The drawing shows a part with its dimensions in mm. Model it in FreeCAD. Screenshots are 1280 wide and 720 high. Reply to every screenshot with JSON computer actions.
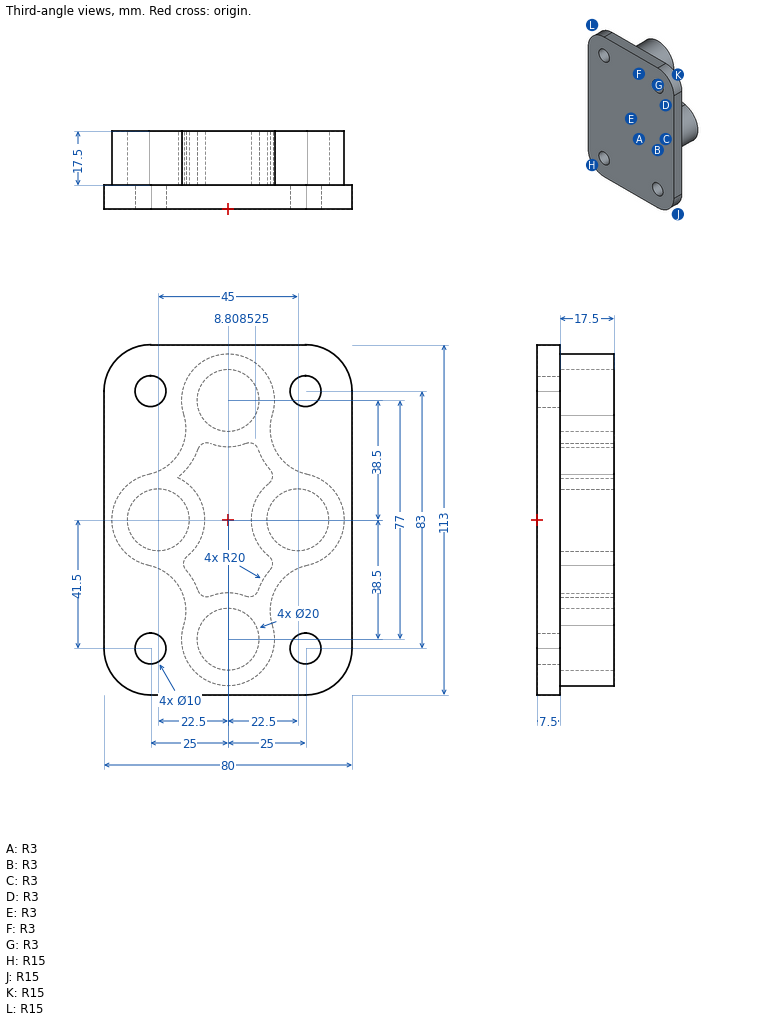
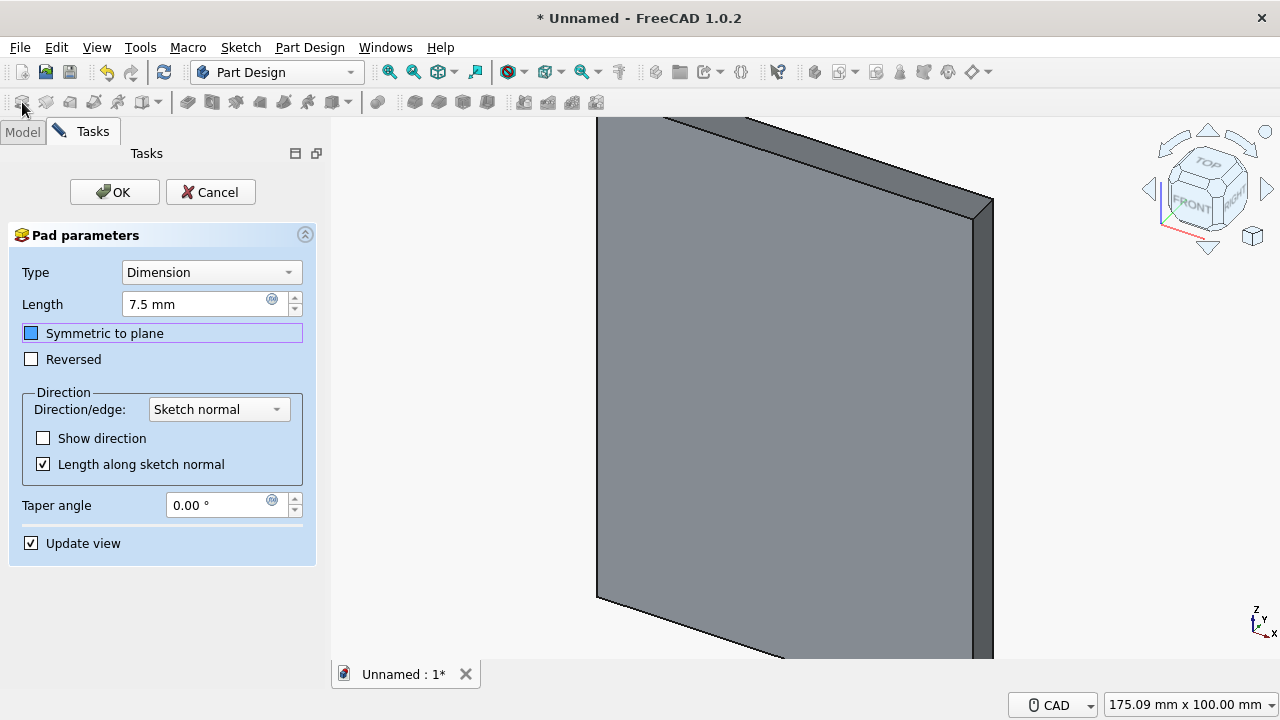
{"action": "left_click", "coordinate": [30, 359]}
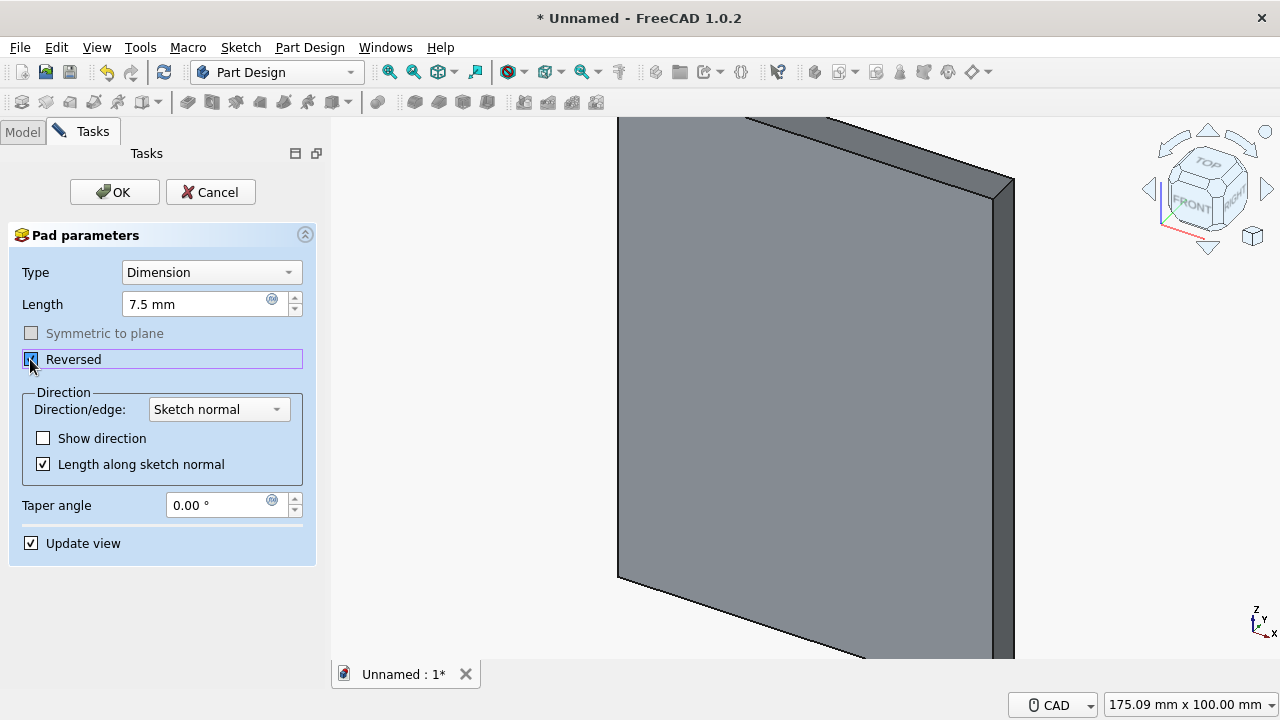
{"action": "left_click", "coordinate": [115, 192]}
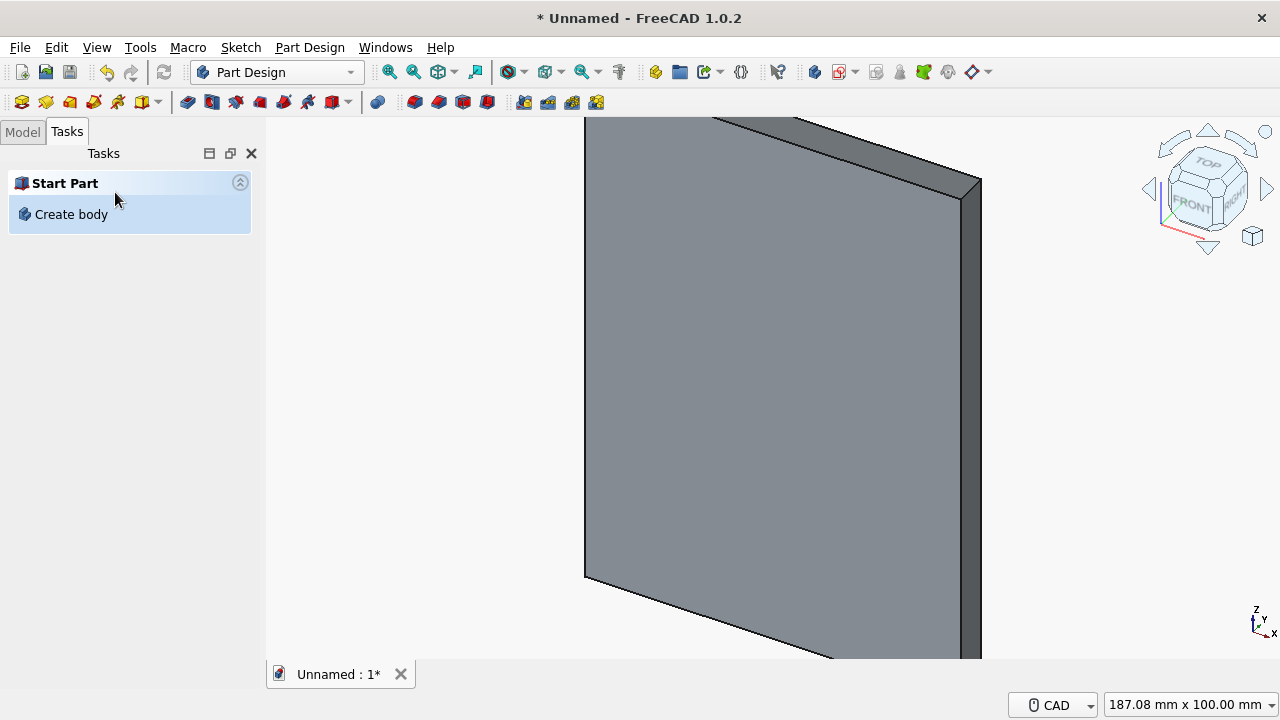
{"action": "key", "text": "v f"}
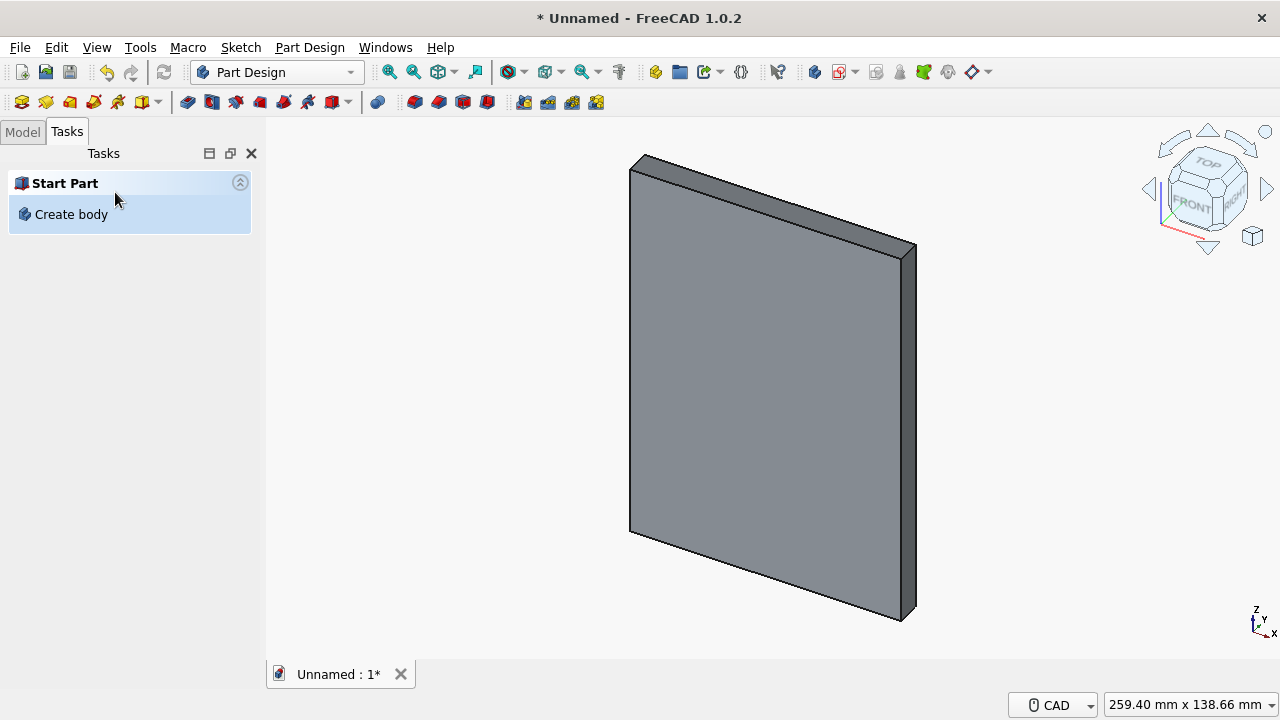
{"action": "key", "text": "4"}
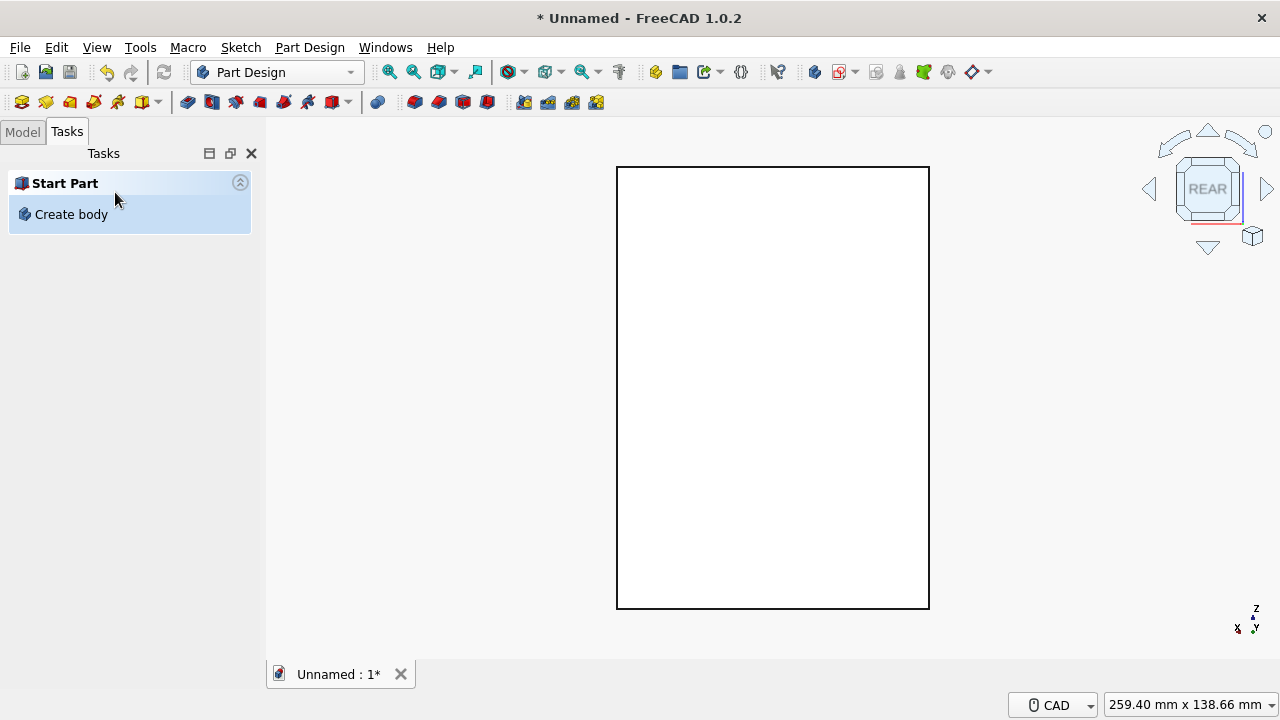
{"action": "left_click", "coordinate": [773, 324]}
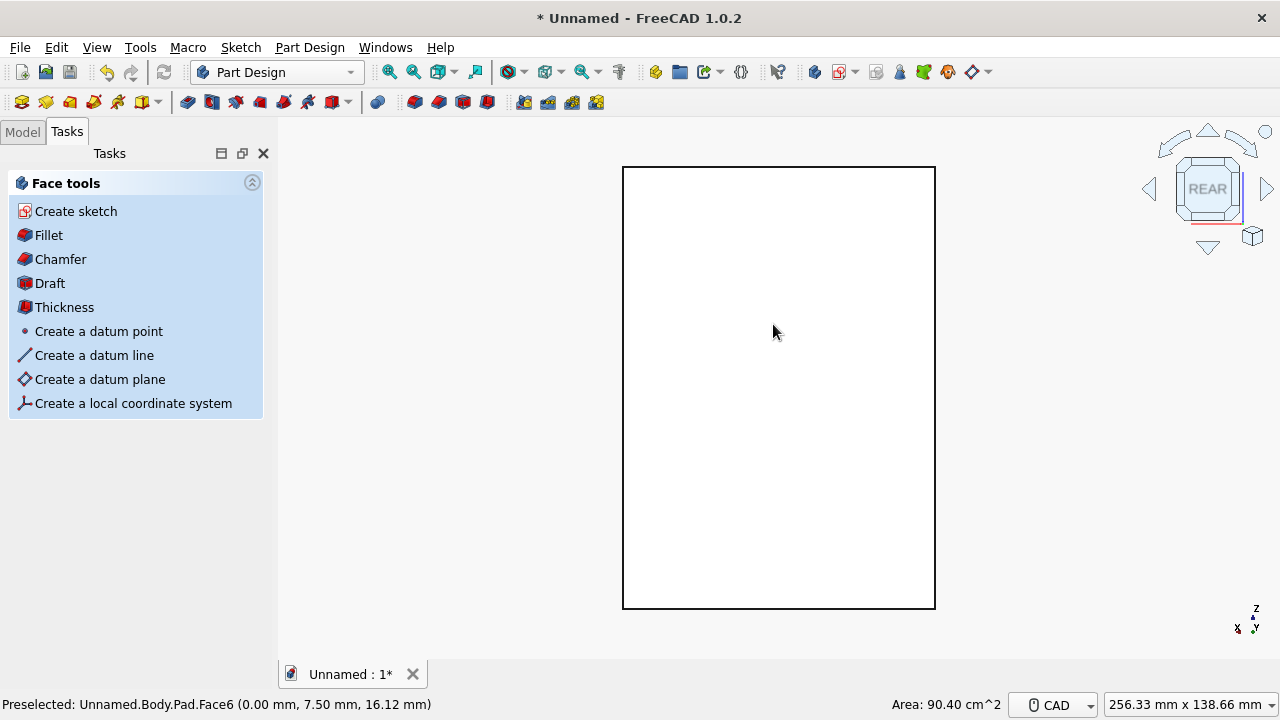
{"action": "left_click", "coordinate": [840, 72]}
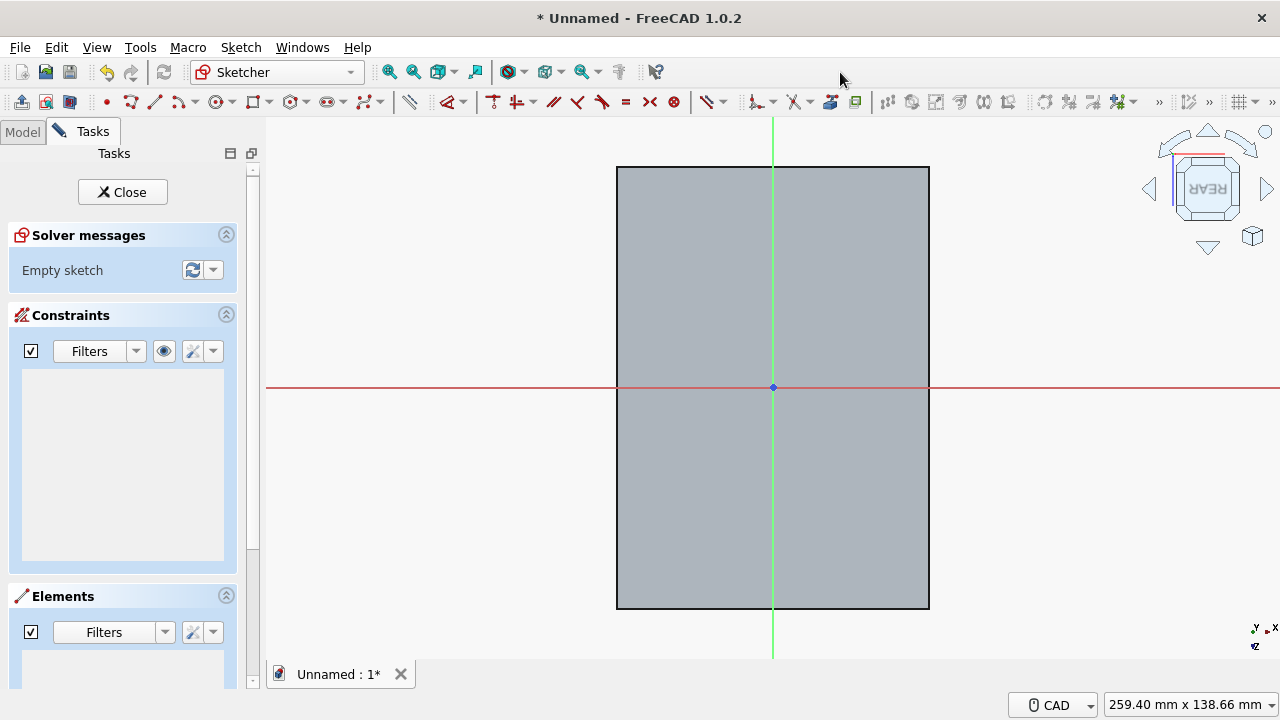
{"action": "key", "text": "g 3 a"}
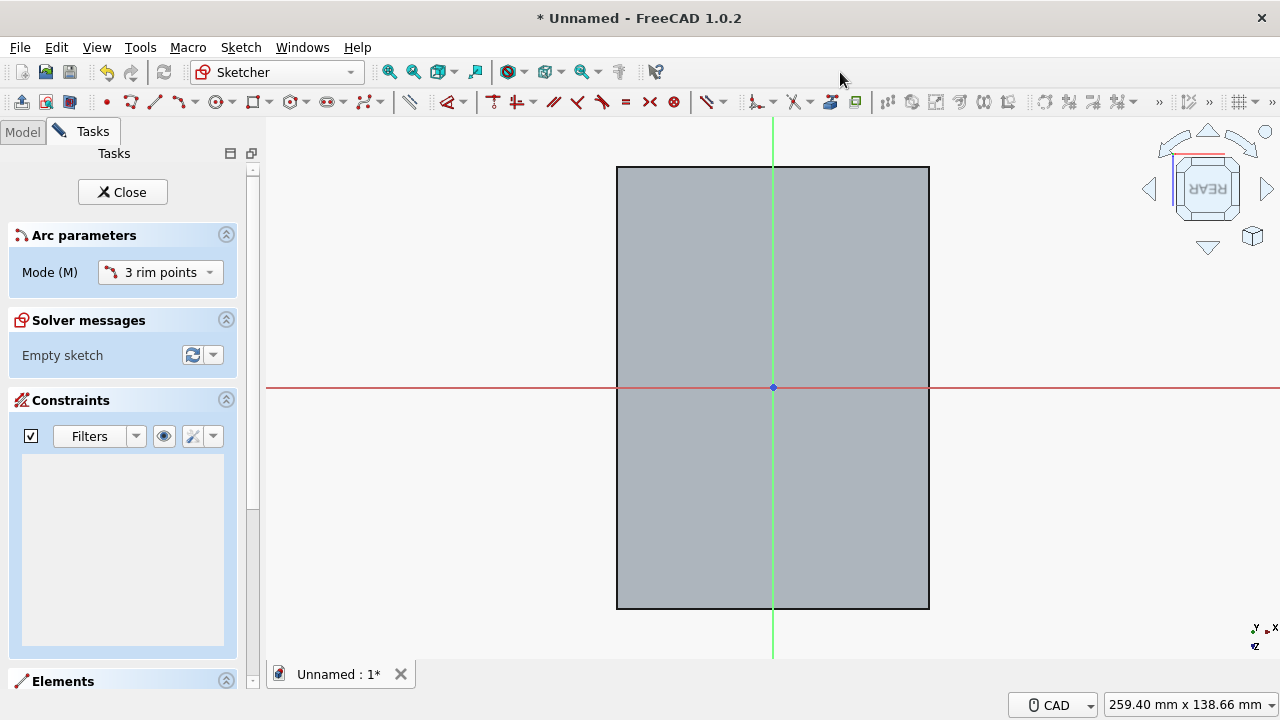
{"action": "left_click", "coordinate": [673, 331]}
{"action": "left_click", "coordinate": [673, 445]}
{"action": "left_click", "coordinate": [629, 372]}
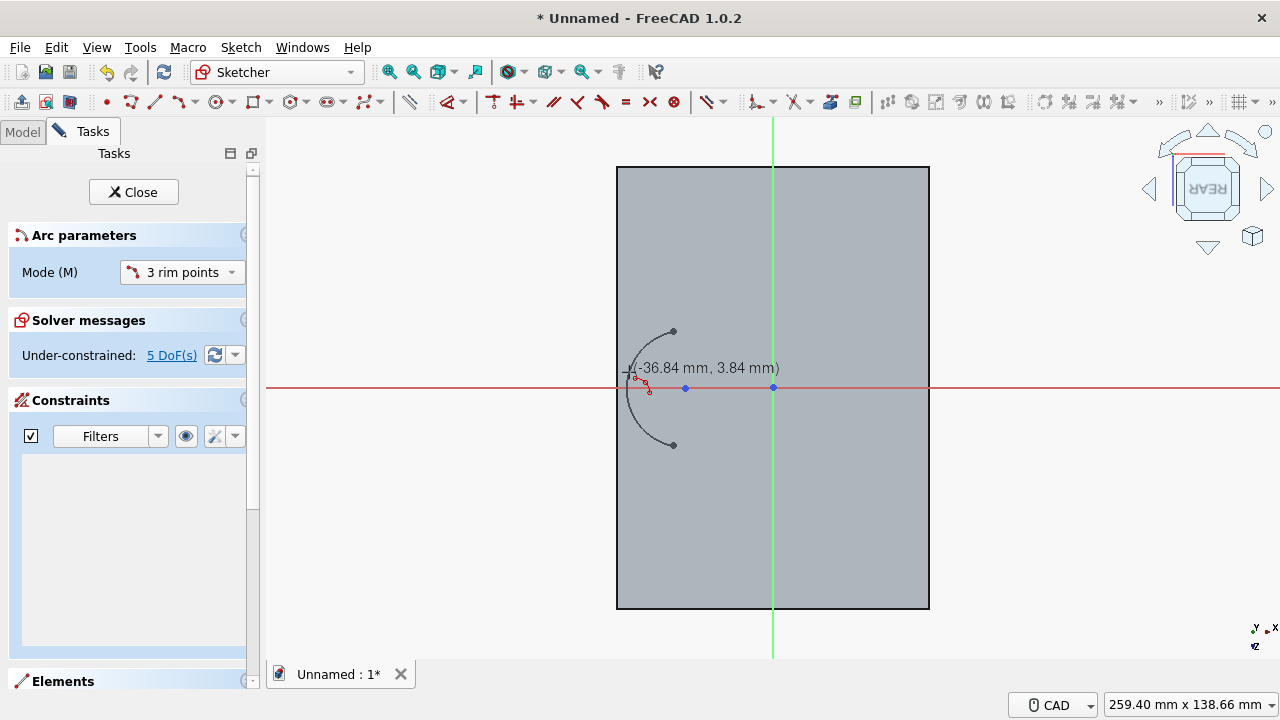
{"action": "left_click", "coordinate": [673, 446]}
{"action": "left_click", "coordinate": [717, 521]}
{"action": "left_click", "coordinate": [712, 473]}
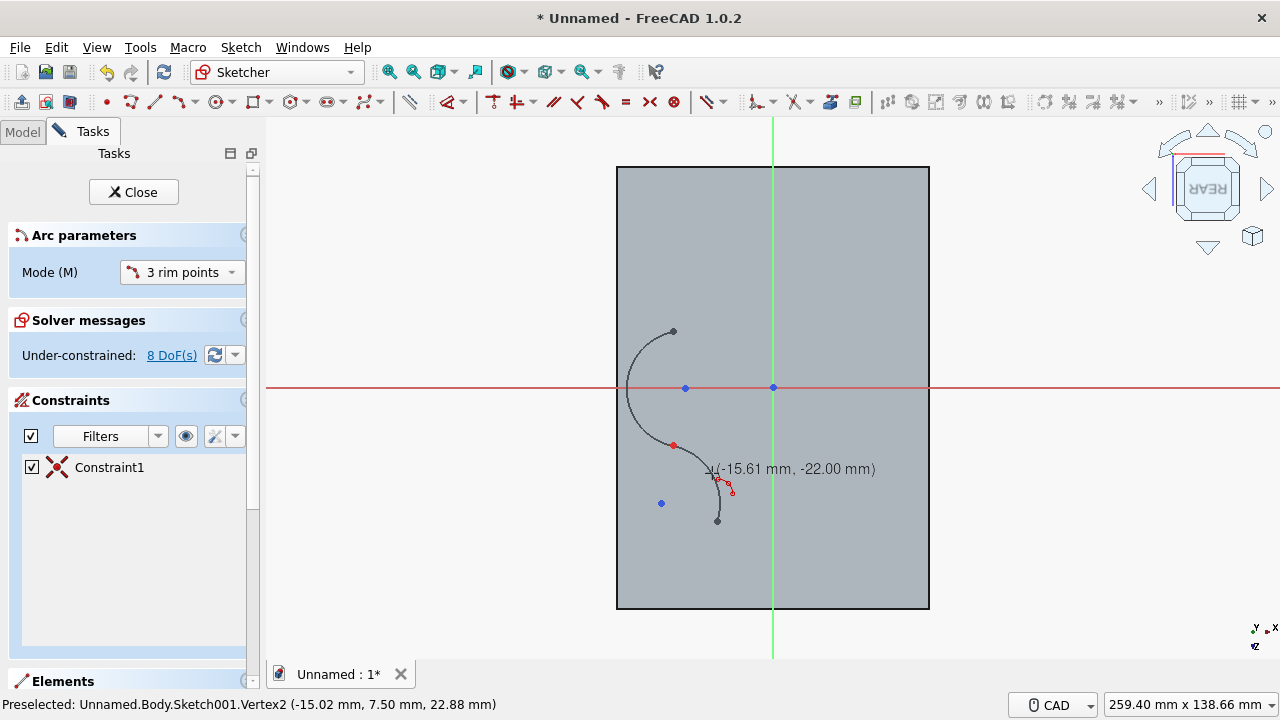
{"action": "left_click", "coordinate": [717, 522]}
{"action": "left_click", "coordinate": [829, 521]}
{"action": "left_click", "coordinate": [751, 593]}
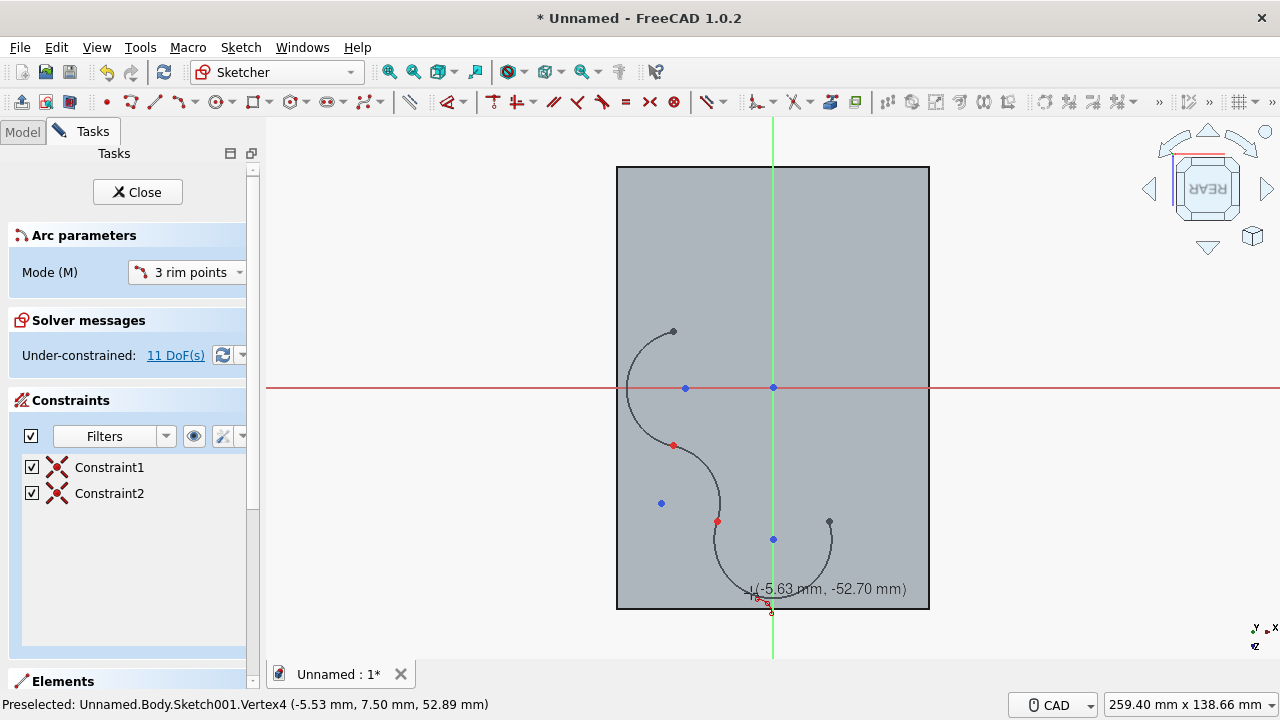
{"action": "left_click", "coordinate": [829, 522]}
{"action": "left_click", "coordinate": [873, 445]}
{"action": "left_click", "coordinate": [834, 473]}